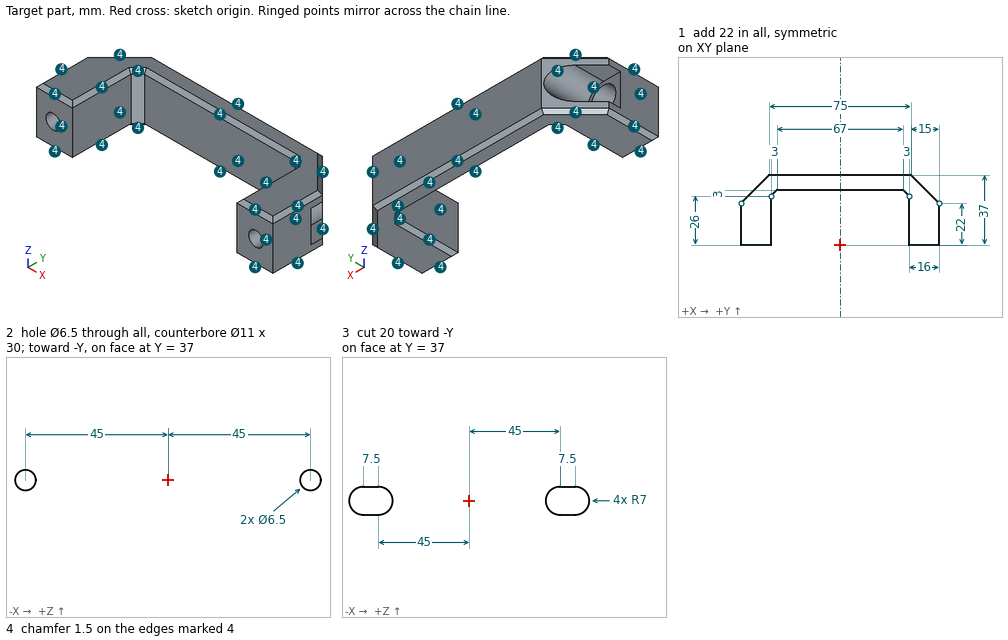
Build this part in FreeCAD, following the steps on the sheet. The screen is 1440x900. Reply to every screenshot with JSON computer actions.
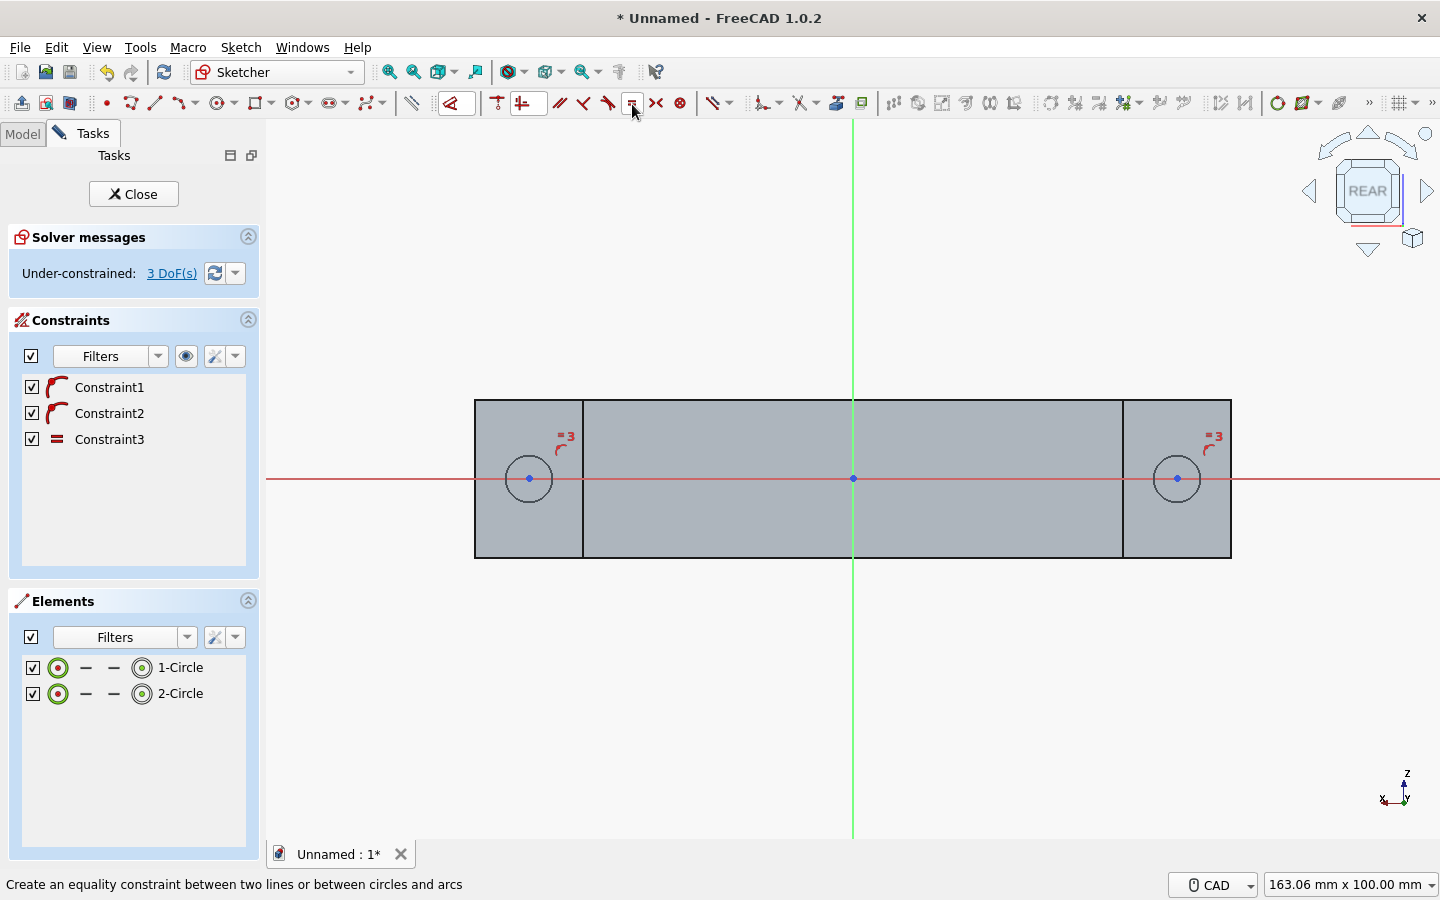
{"action": "left_click", "coordinate": [1193, 462]}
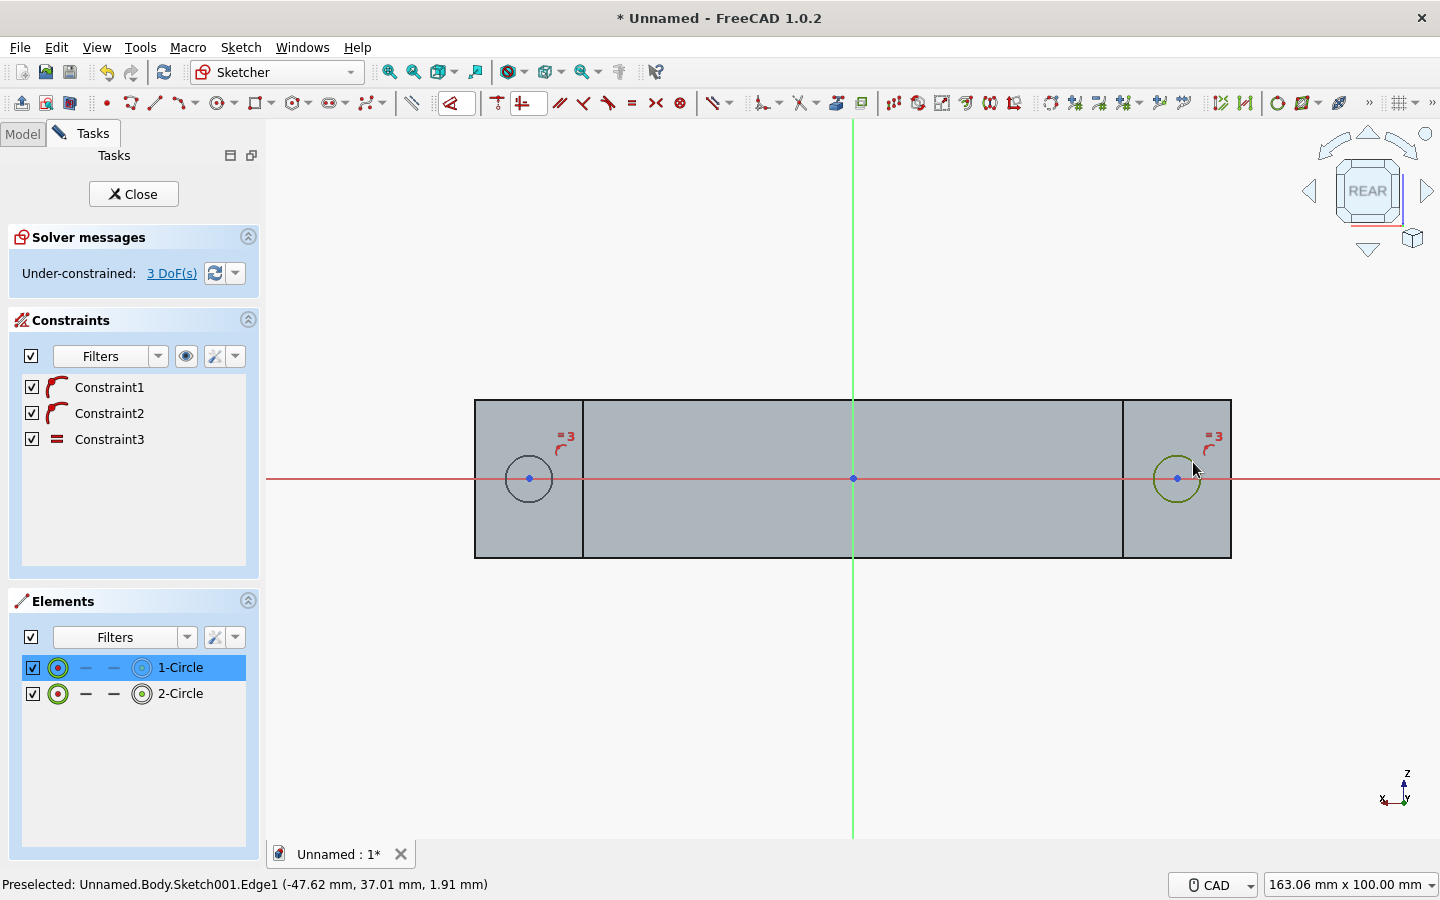
{"action": "key", "text": "k o"}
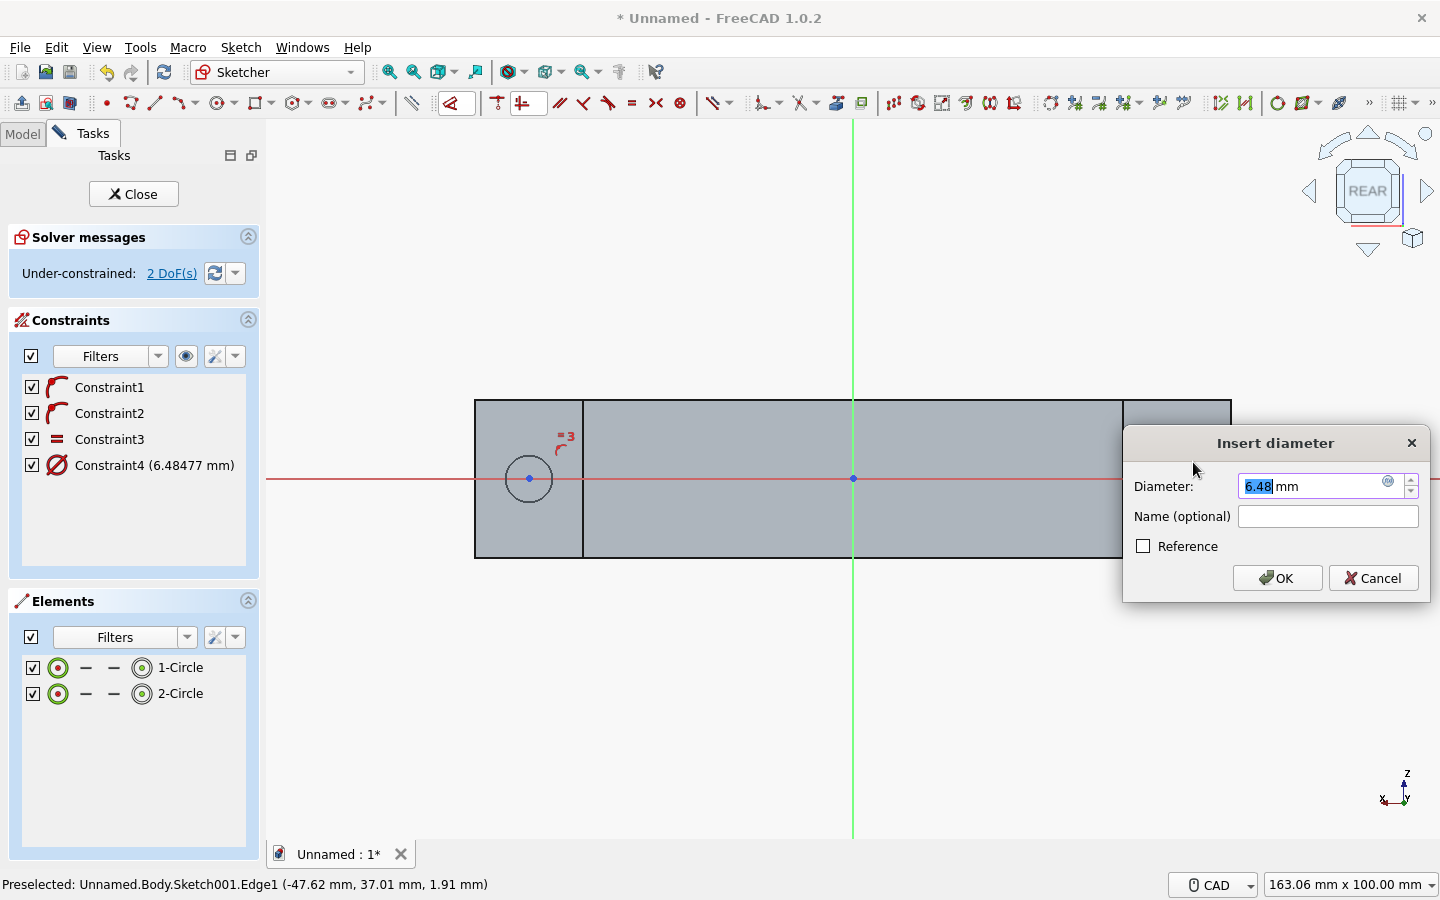
{"action": "type", "text": "6.5"}
{"action": "key", "text": "Return"}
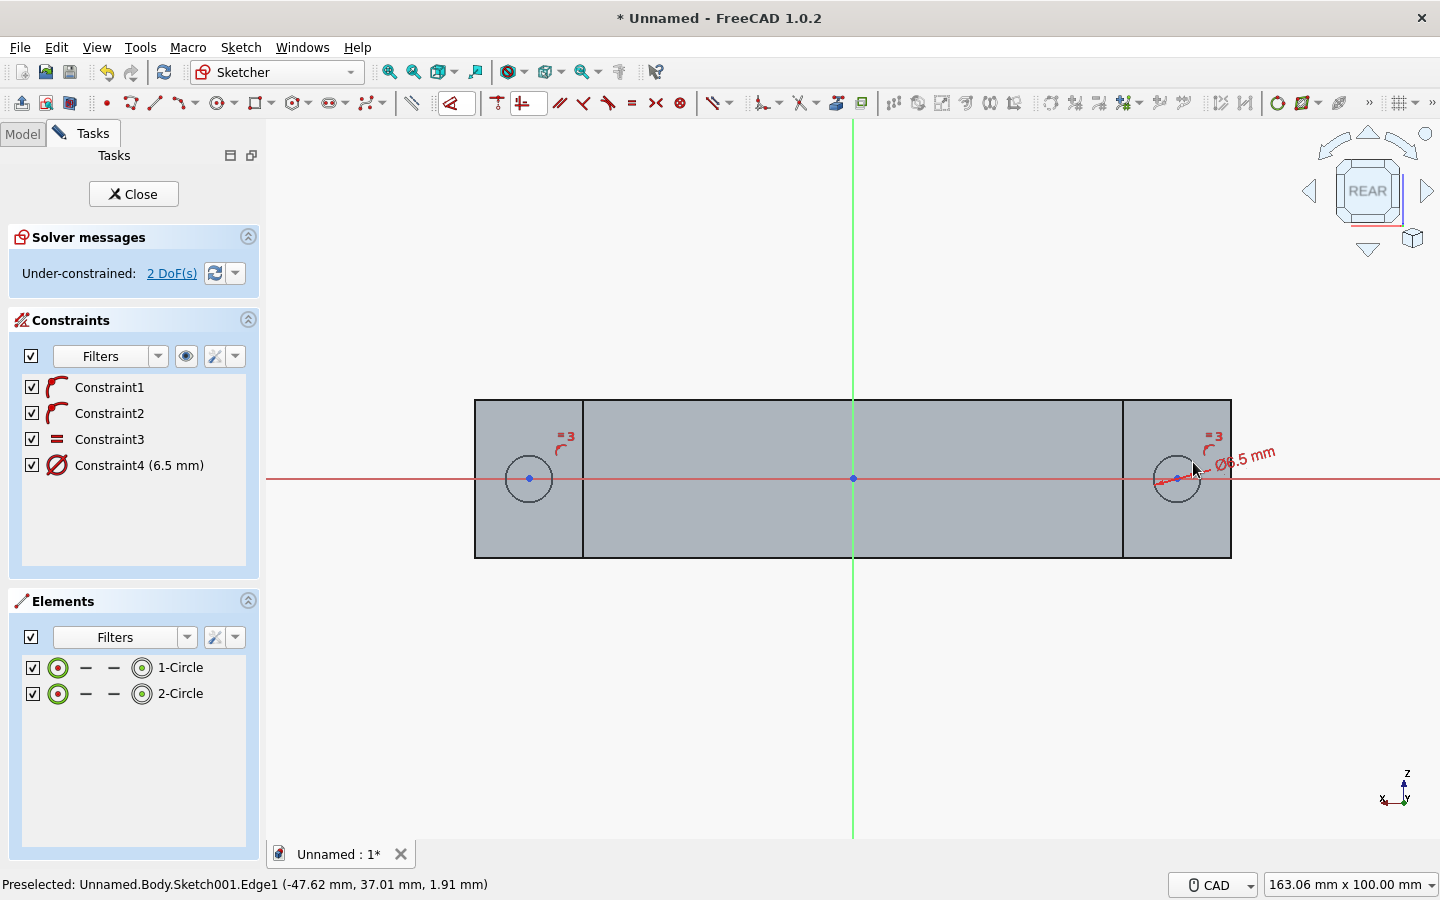
{"action": "left_click", "coordinate": [1177, 479]}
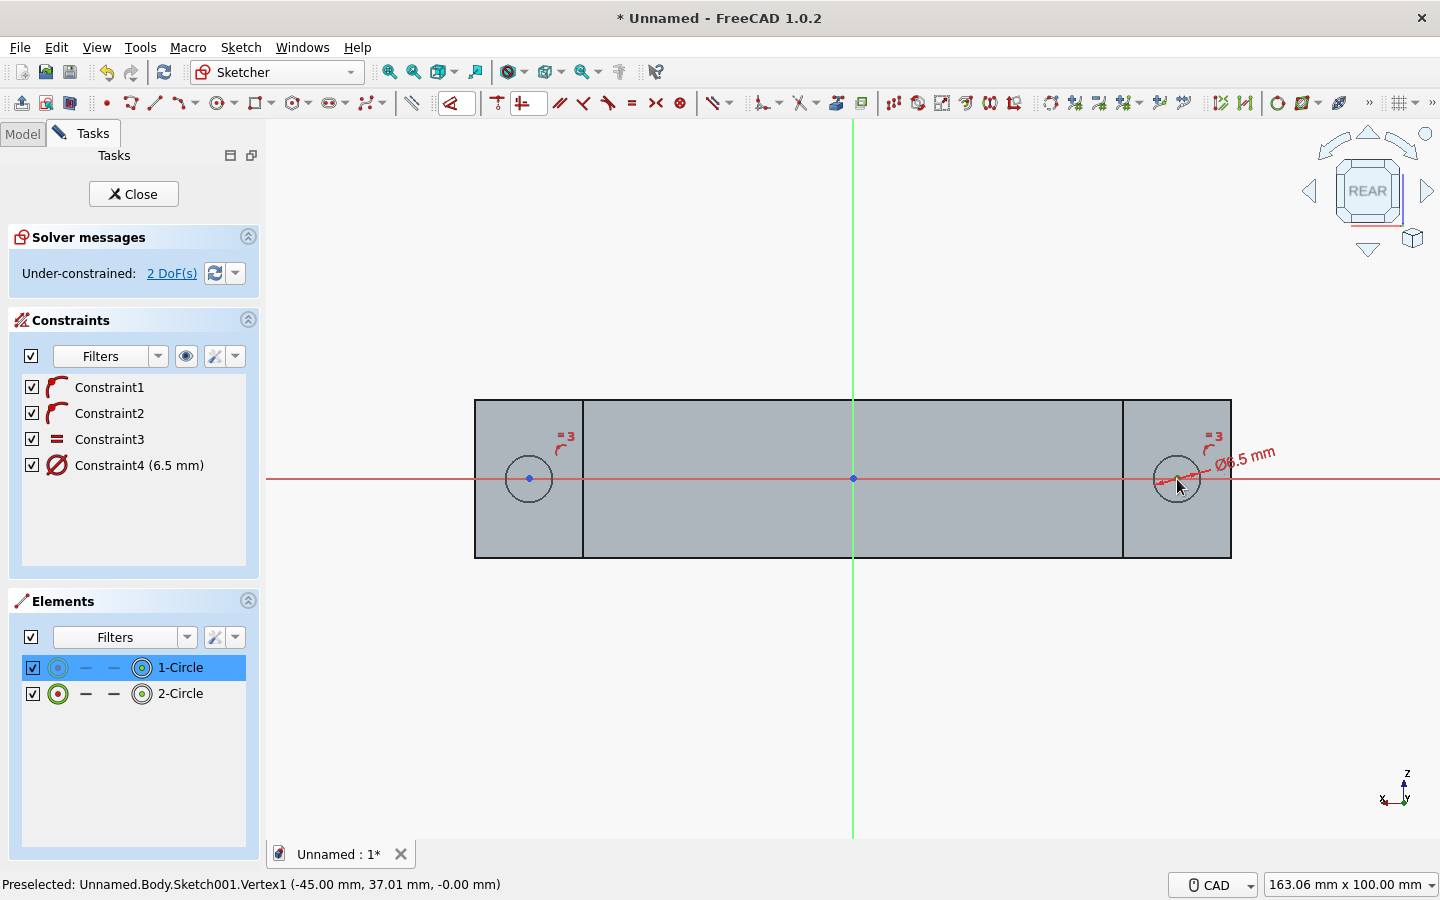
{"action": "left_click", "coordinate": [470, 104]}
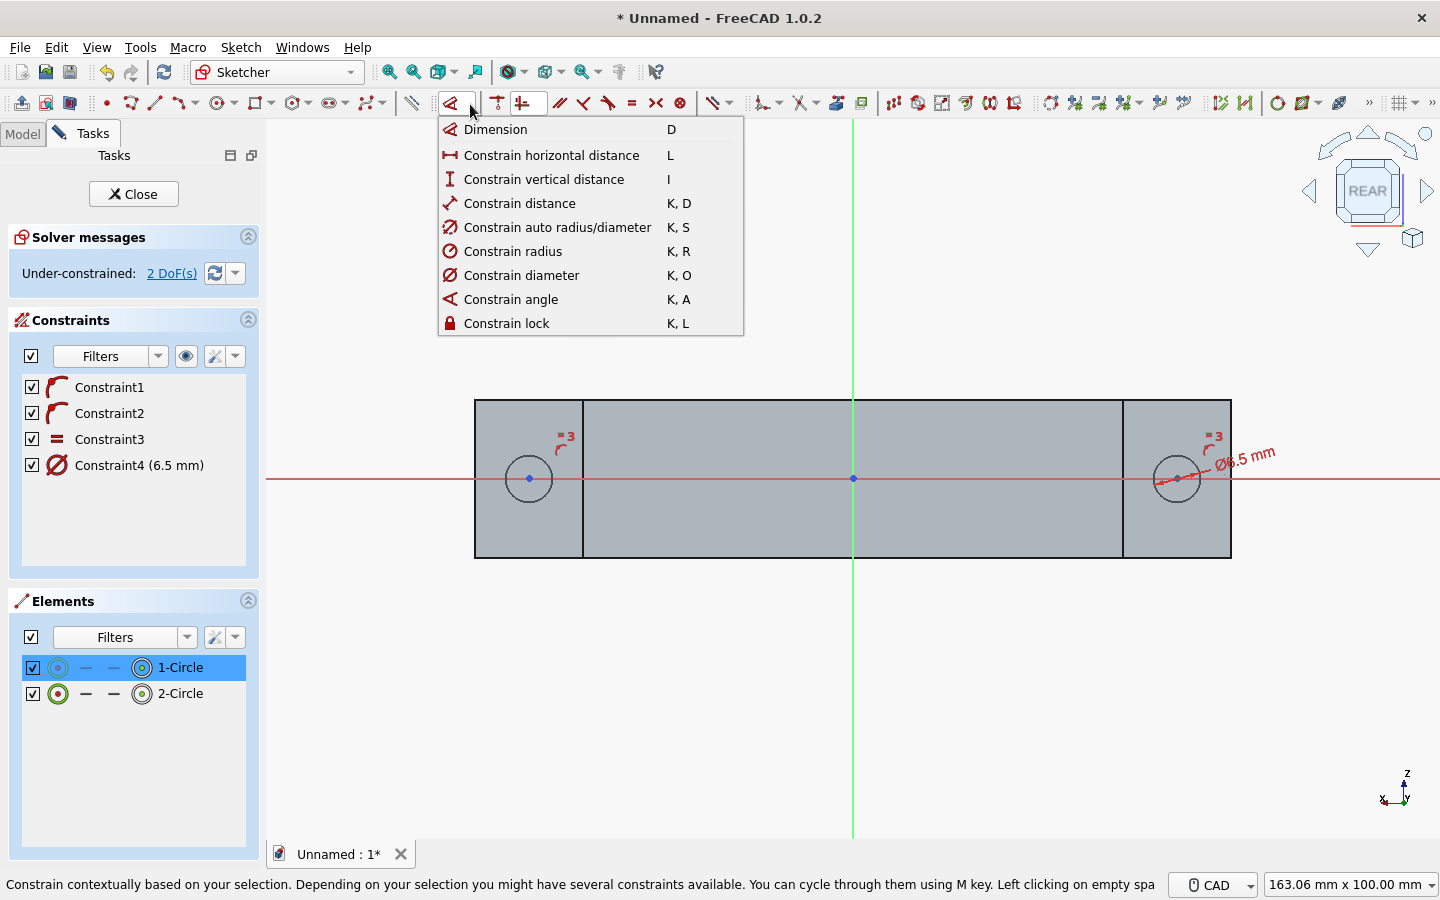
{"action": "left_click", "coordinate": [591, 155]}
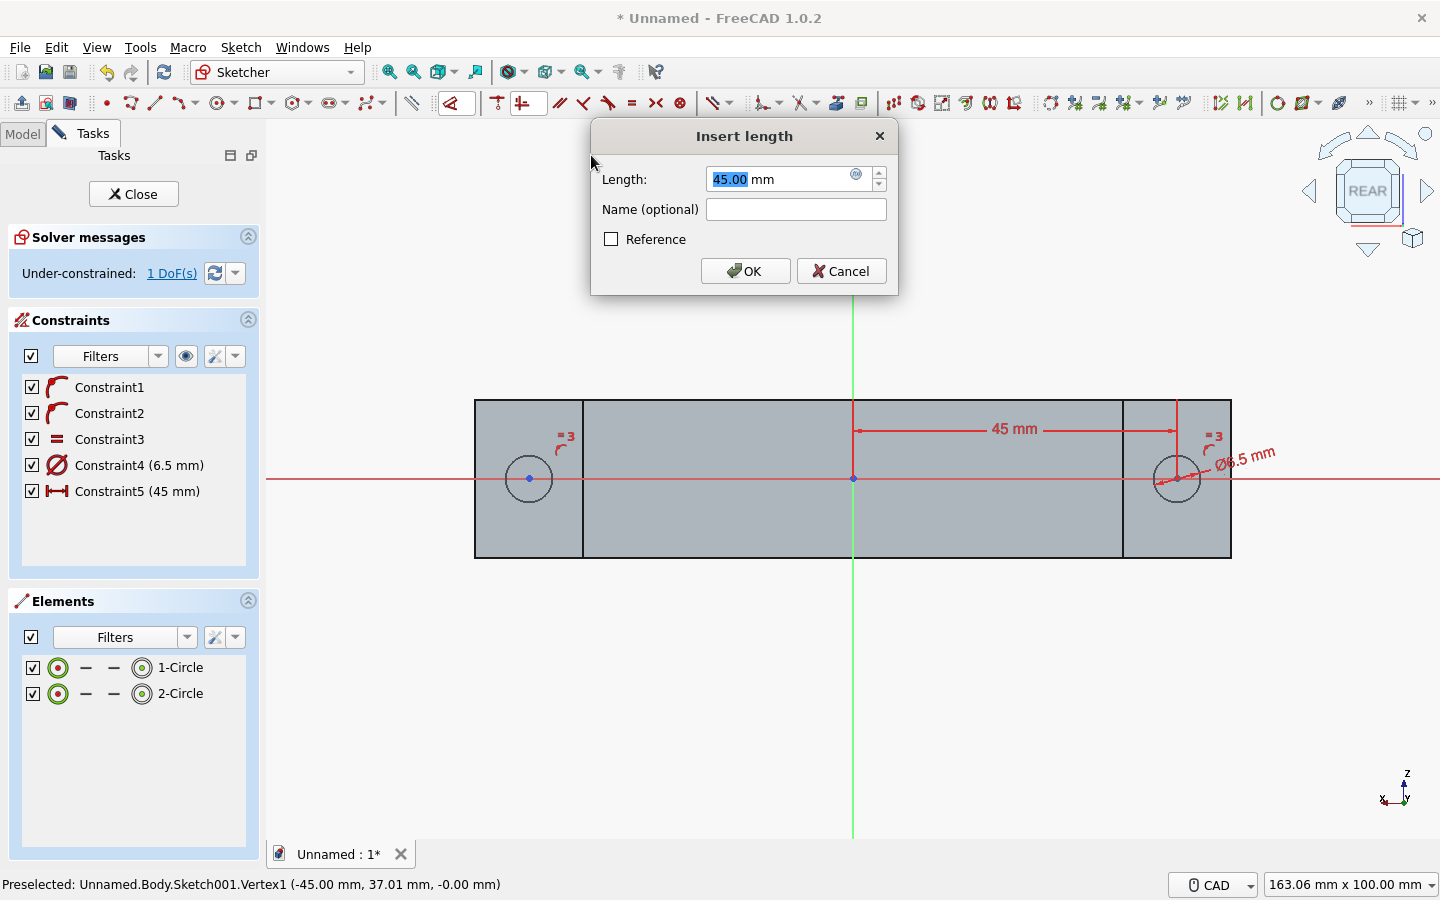
{"action": "type", "text": "45"}
{"action": "key", "text": "Return"}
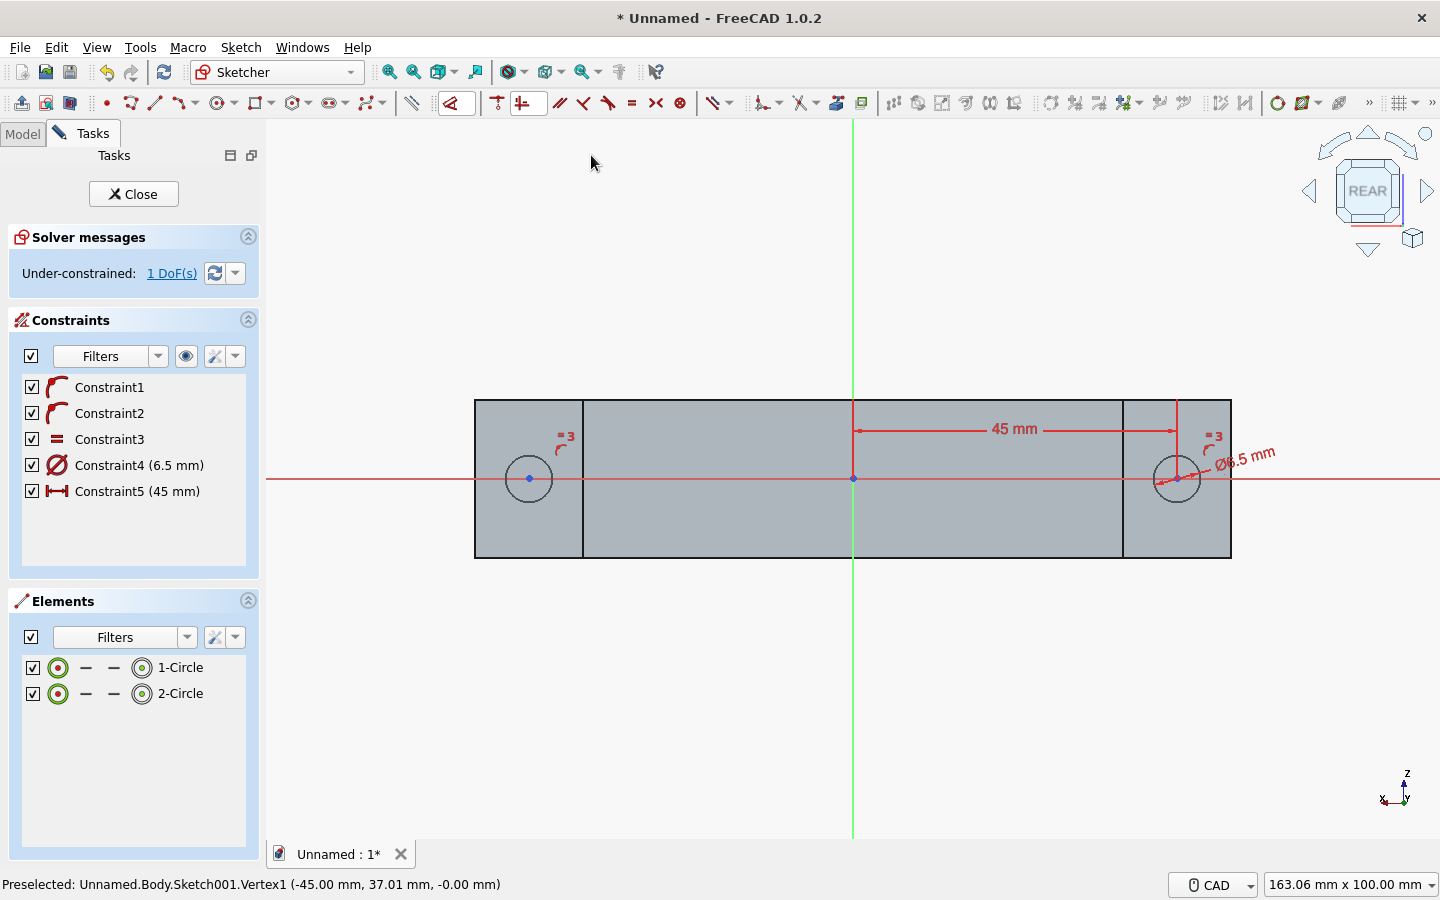
{"action": "left_click", "coordinate": [529, 479]}